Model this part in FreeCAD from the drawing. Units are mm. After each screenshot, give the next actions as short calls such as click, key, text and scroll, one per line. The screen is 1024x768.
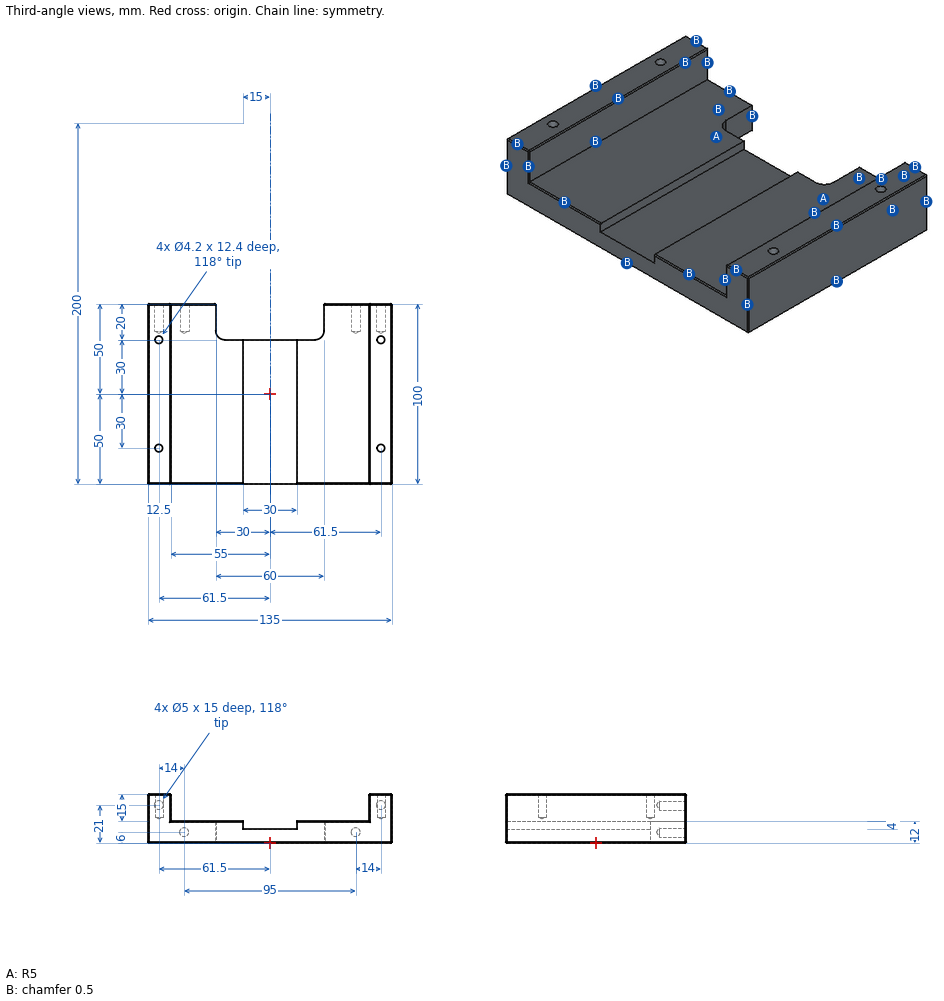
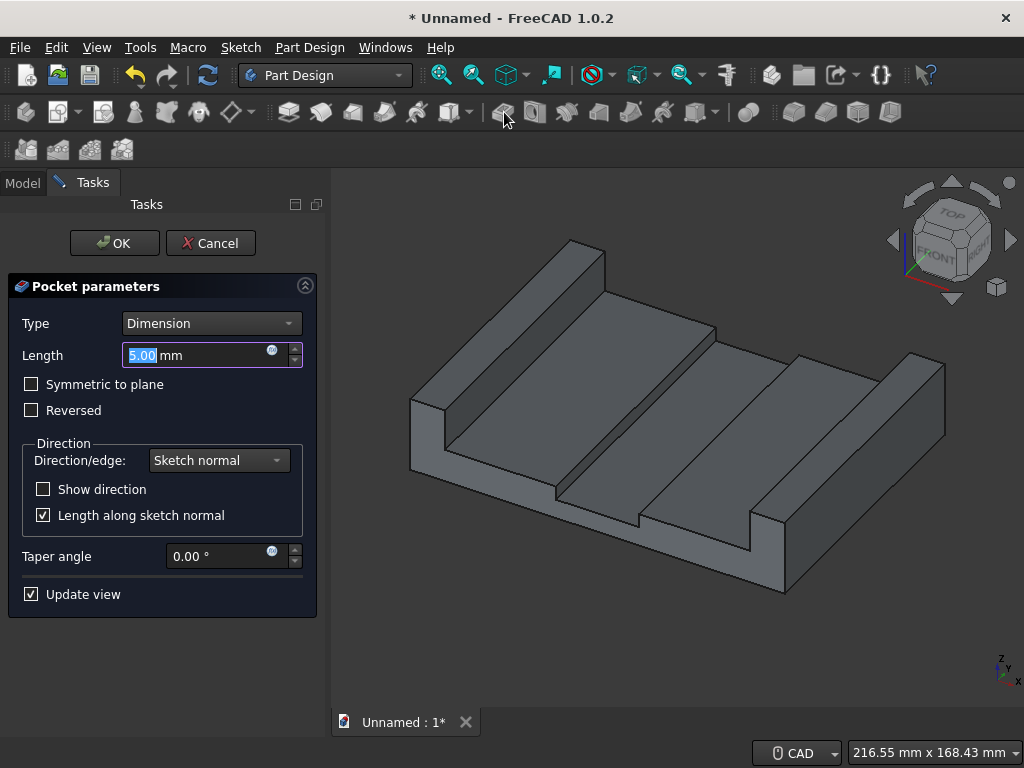
text(4)
key(Tab)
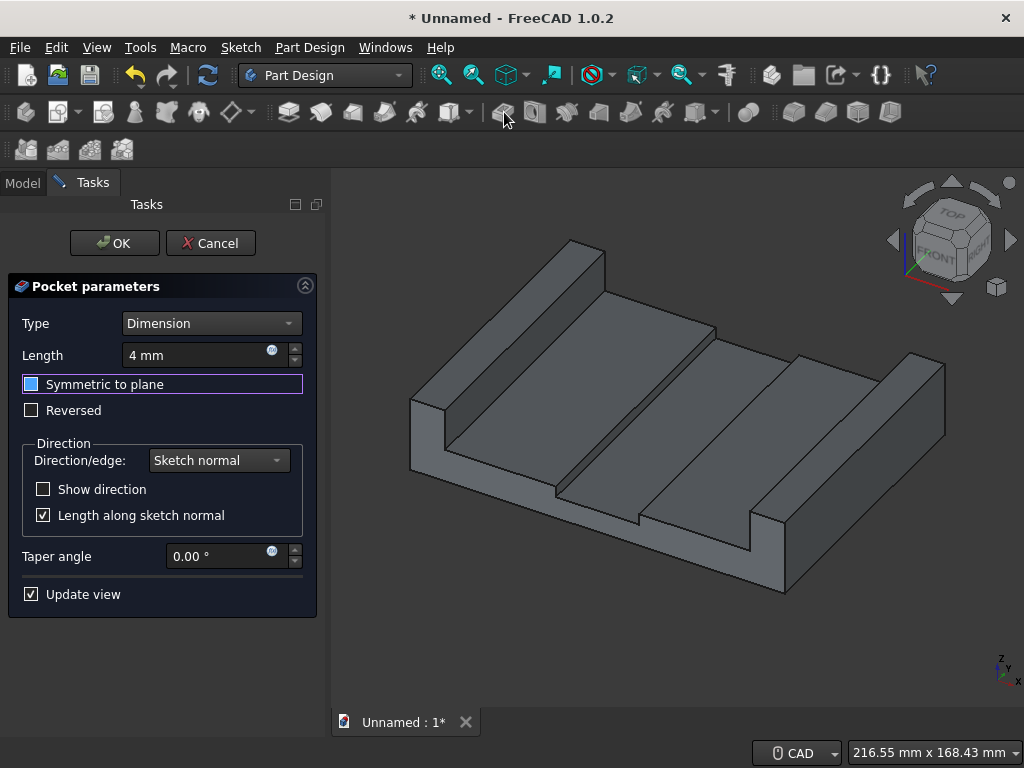
click(115, 243)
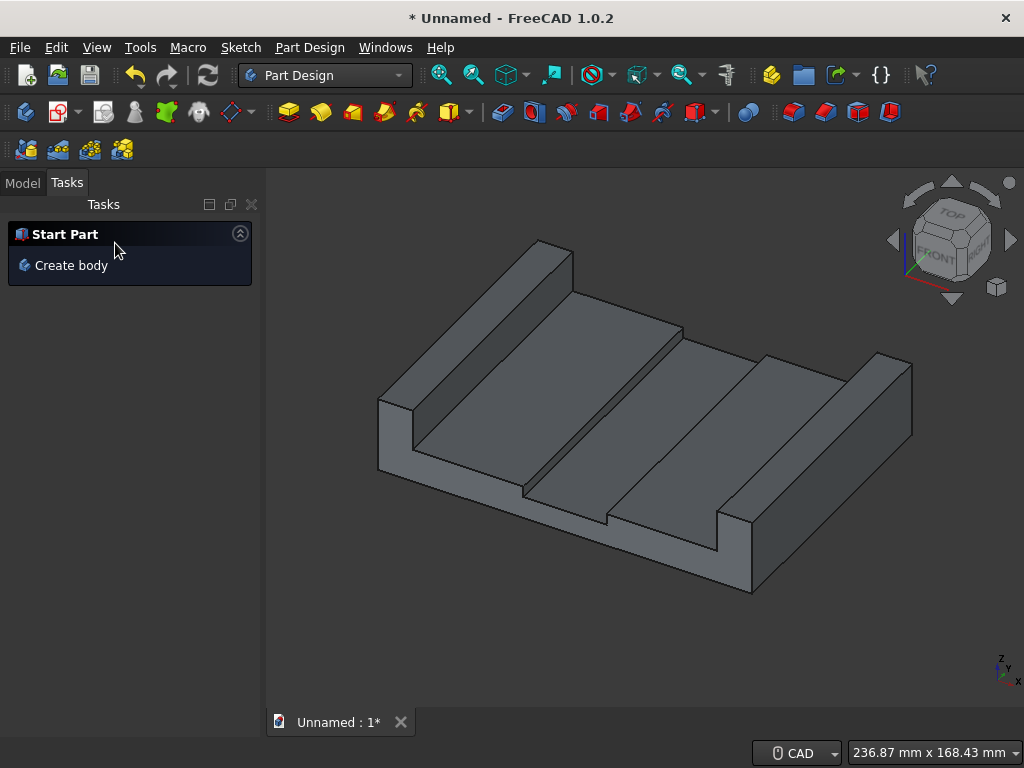
click(594, 342)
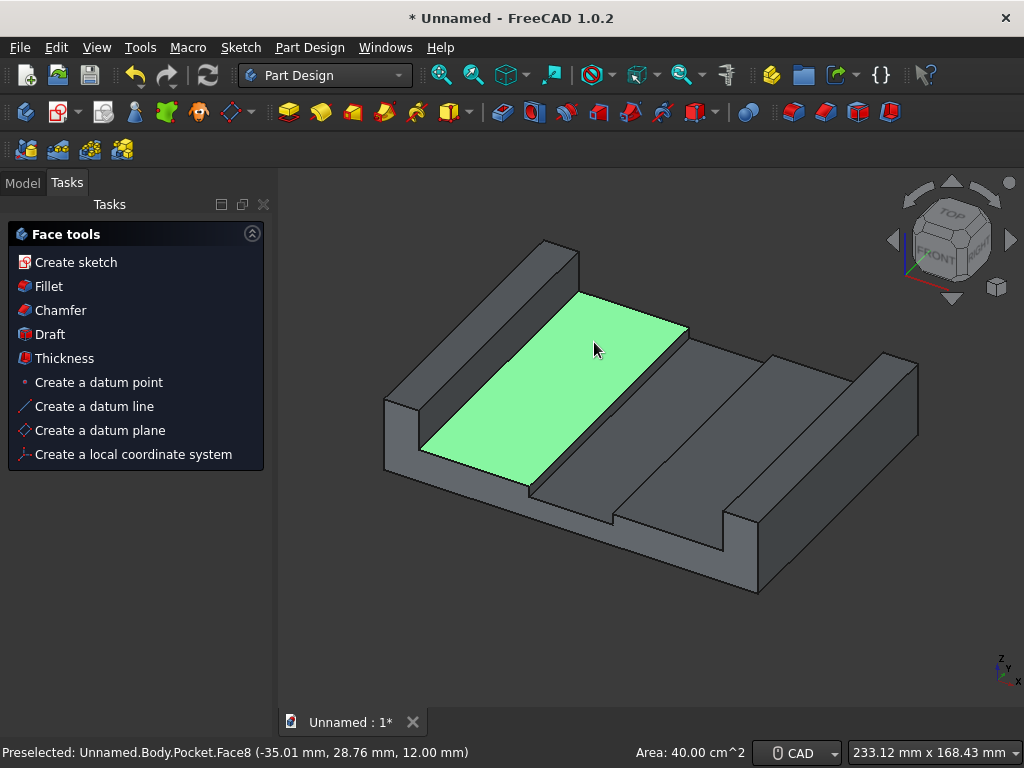
click(58, 112)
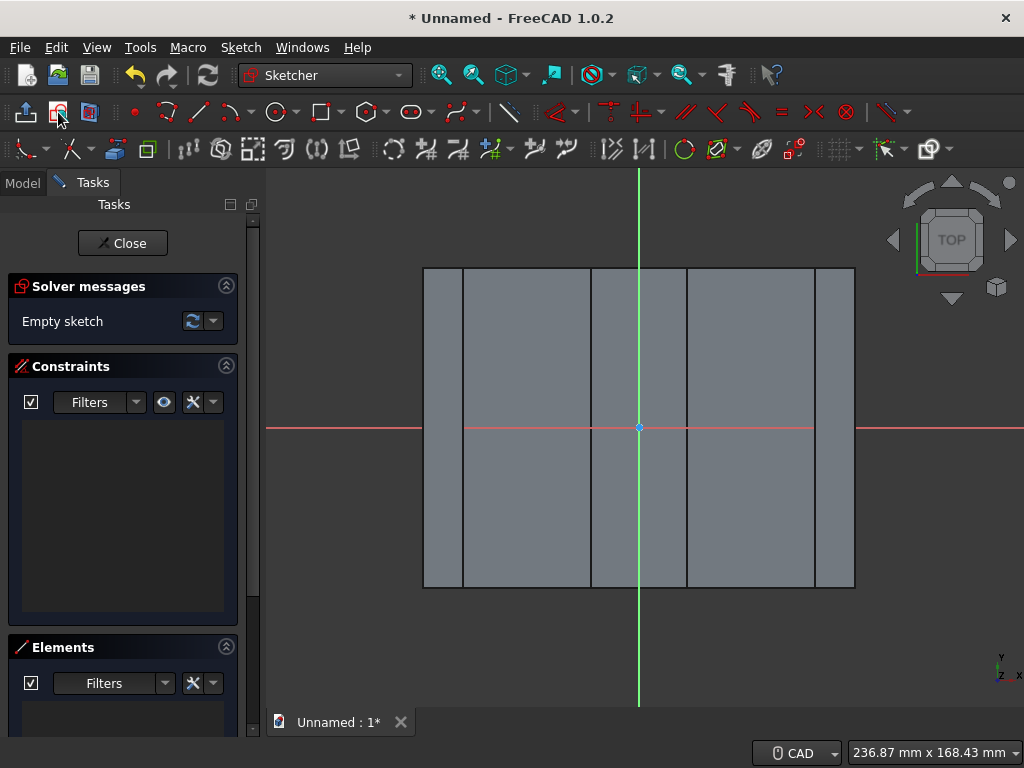
click(90, 112)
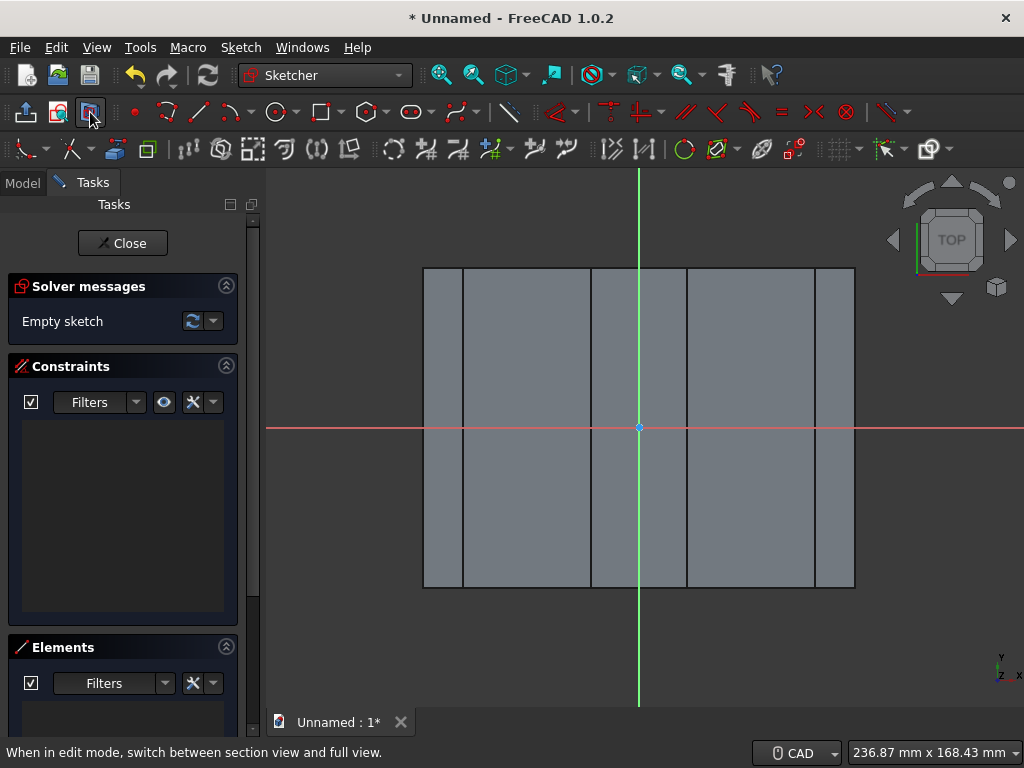
scroll(691, 275, up, 4)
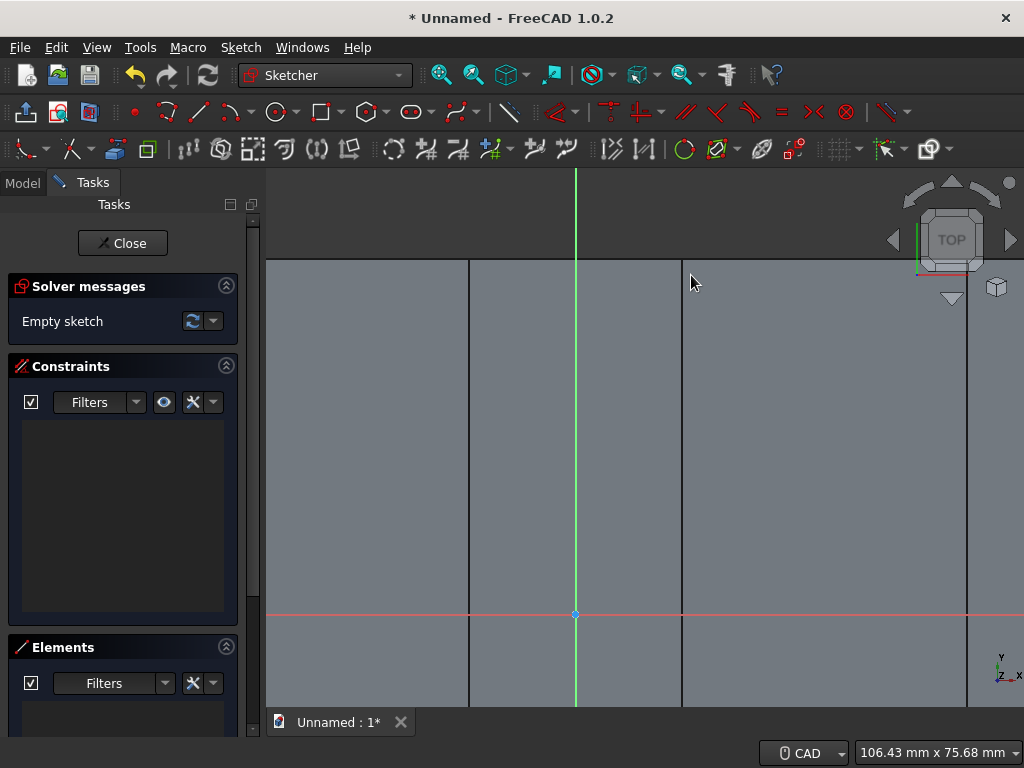
click(322, 112)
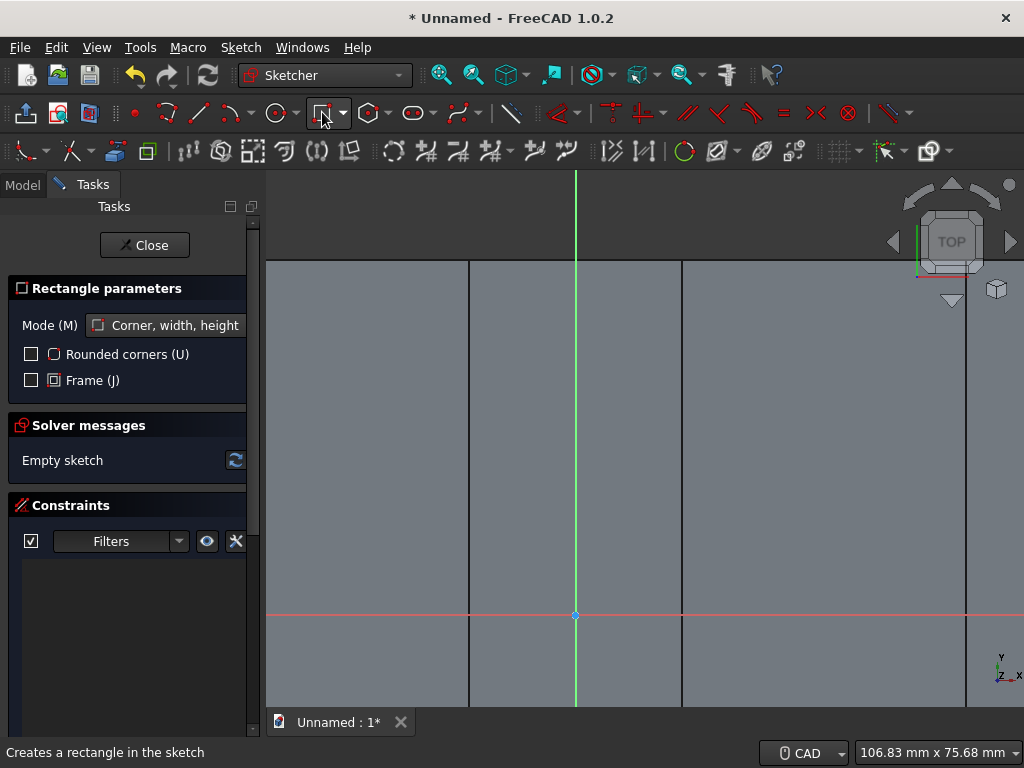
click(363, 260)
click(789, 402)
key(Escape)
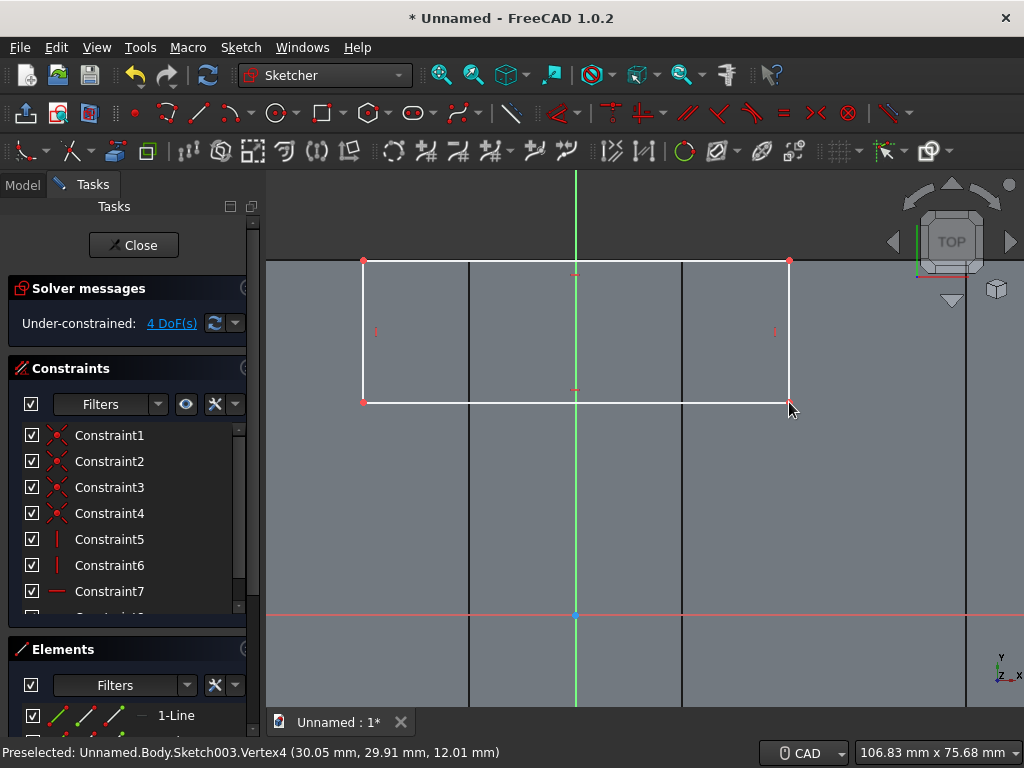
click(558, 114)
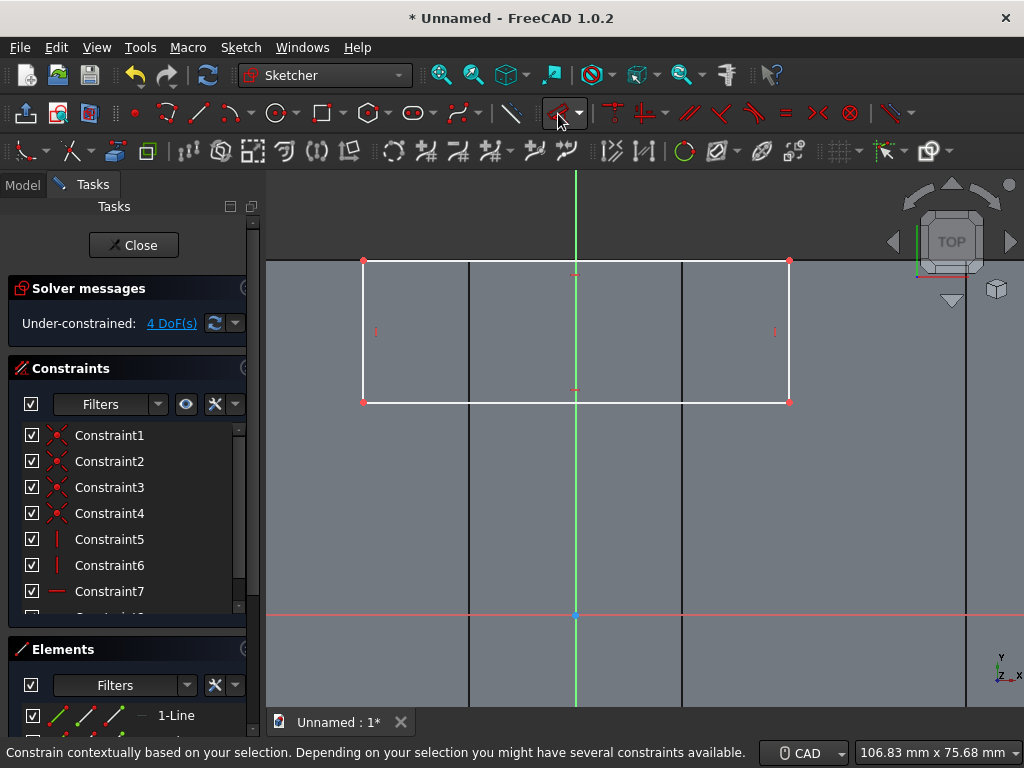
click(363, 304)
click(329, 332)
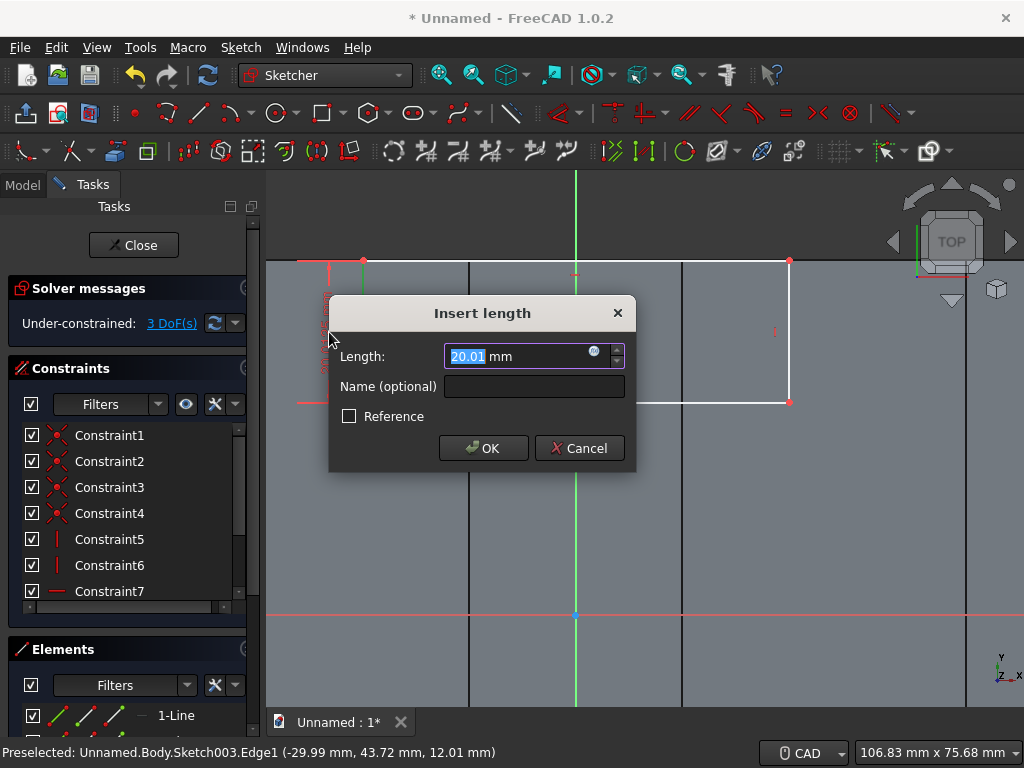
text(20)
key(Return)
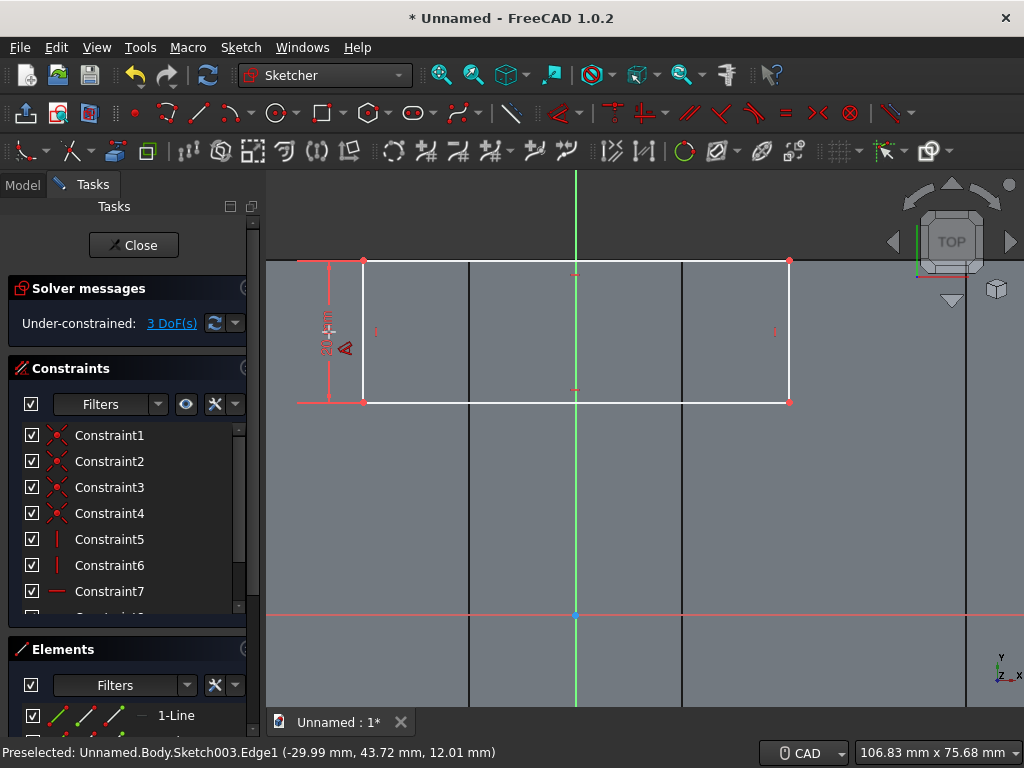
click(491, 403)
click(478, 369)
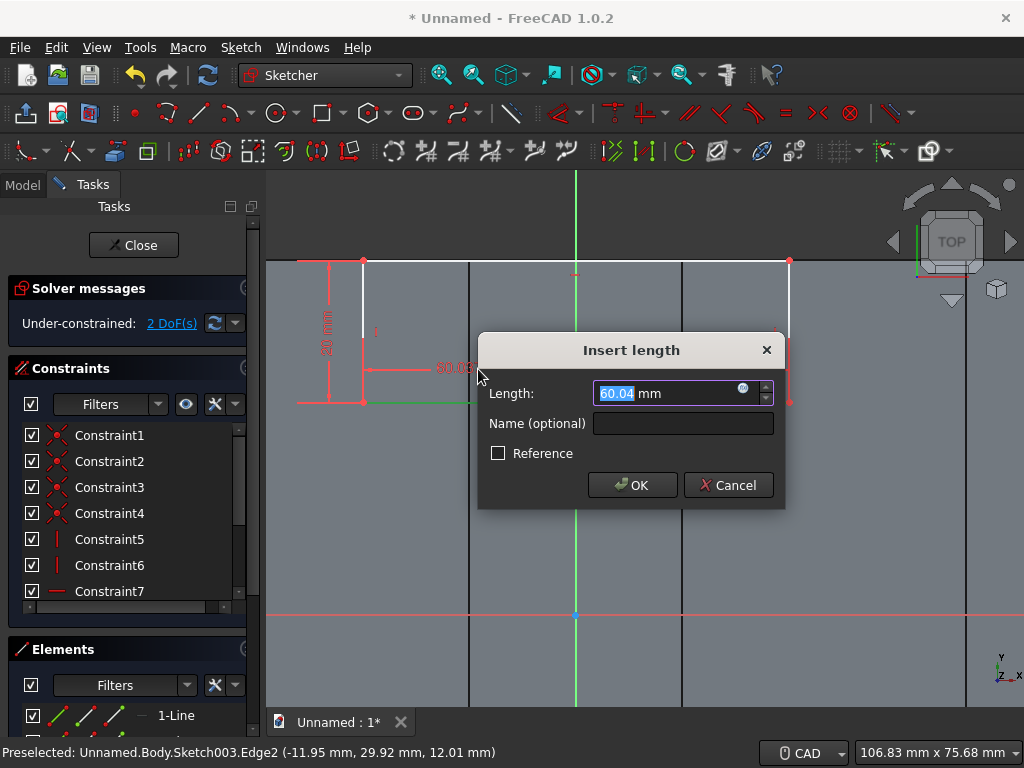
text(60)
key(Return)